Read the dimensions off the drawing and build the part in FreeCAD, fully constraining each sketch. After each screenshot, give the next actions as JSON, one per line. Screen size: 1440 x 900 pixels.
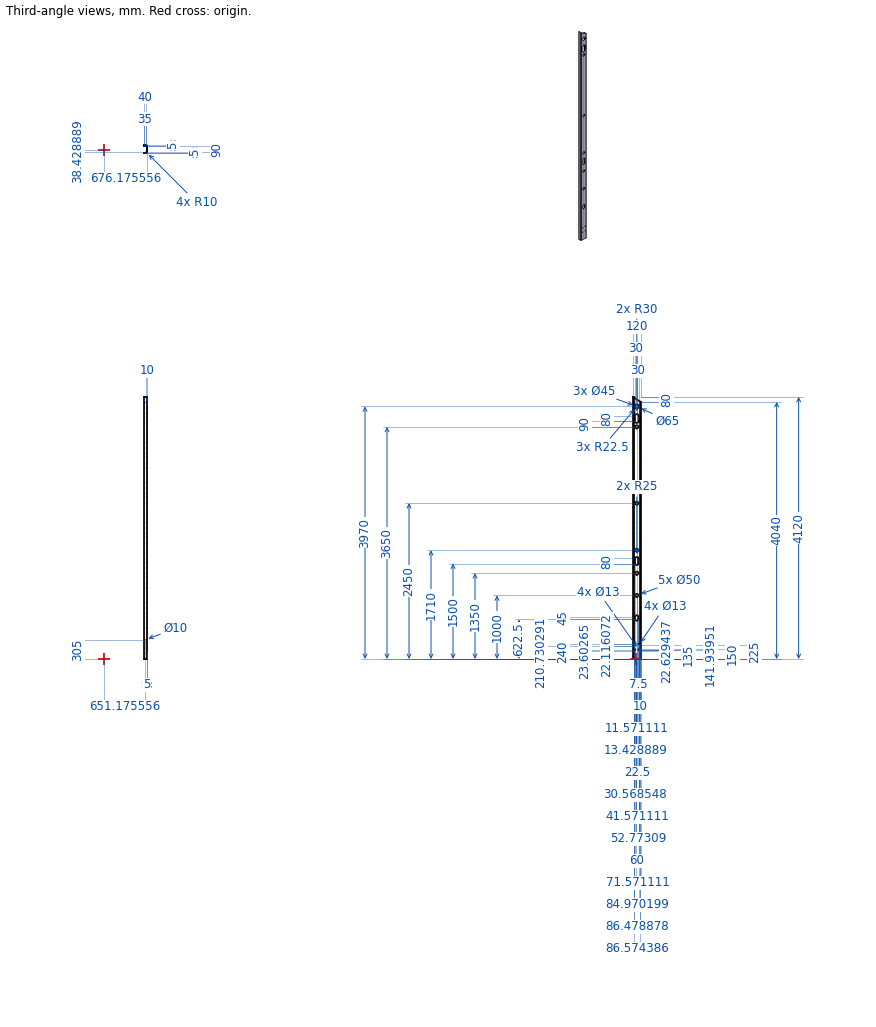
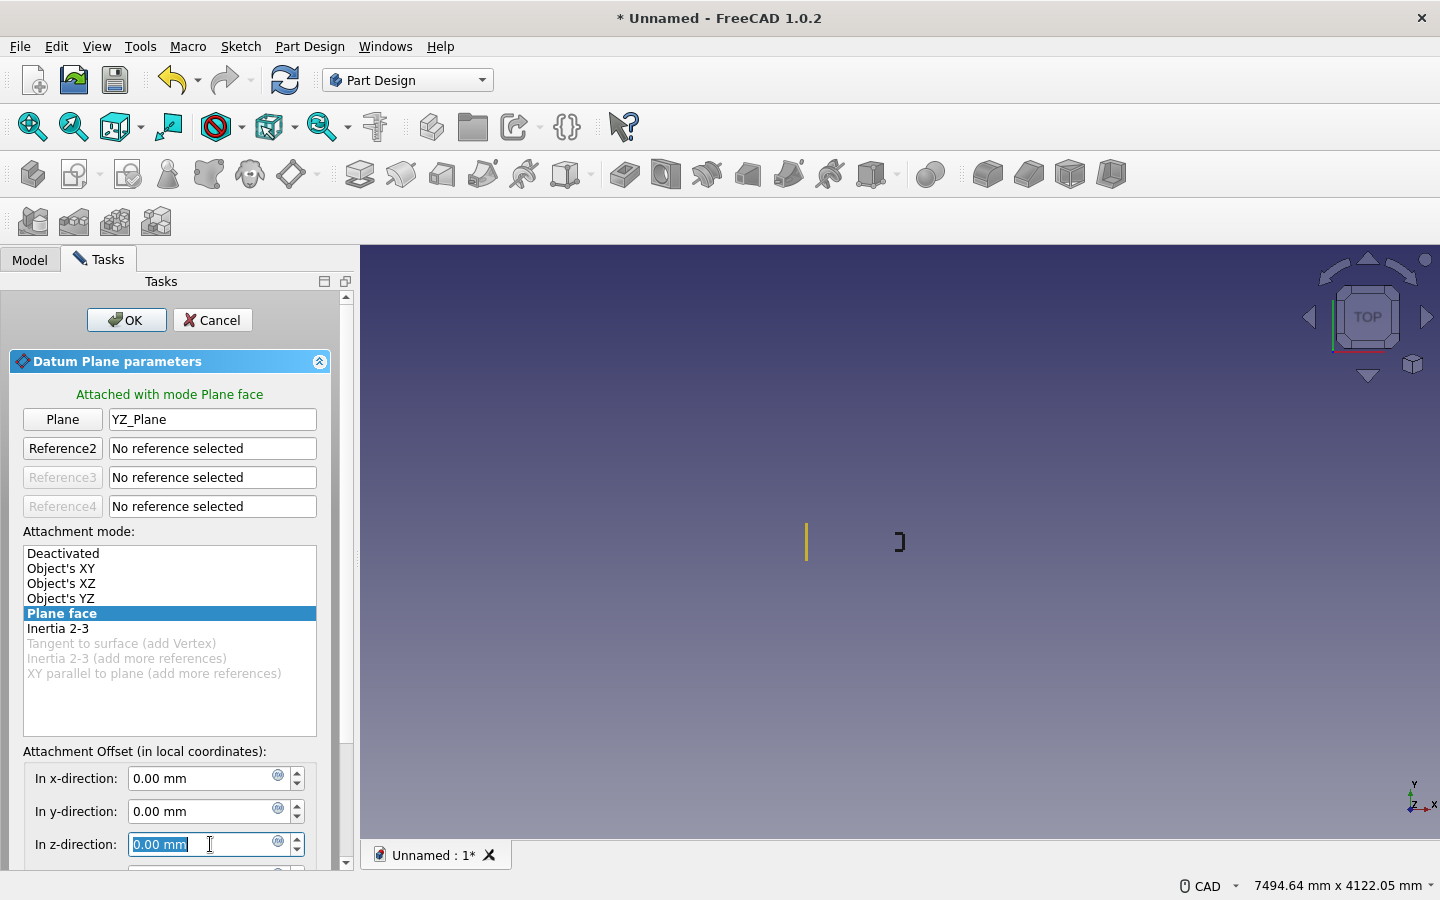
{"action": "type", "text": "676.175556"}
{"action": "key", "text": "Tab"}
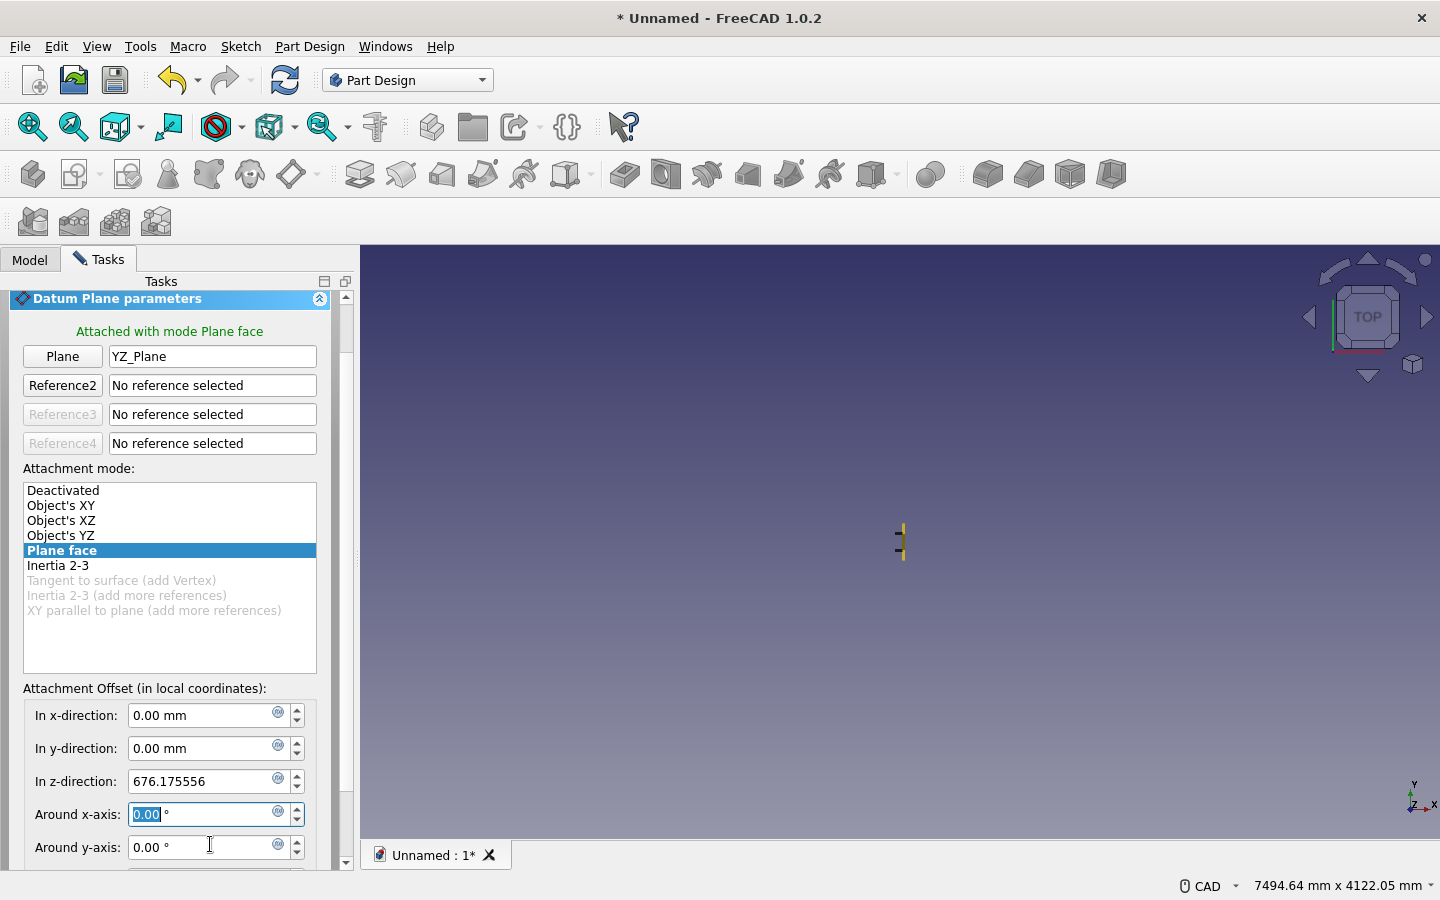
{"action": "scroll", "coordinate": [346, 580], "scroll_direction": "up", "scroll_amount": 2}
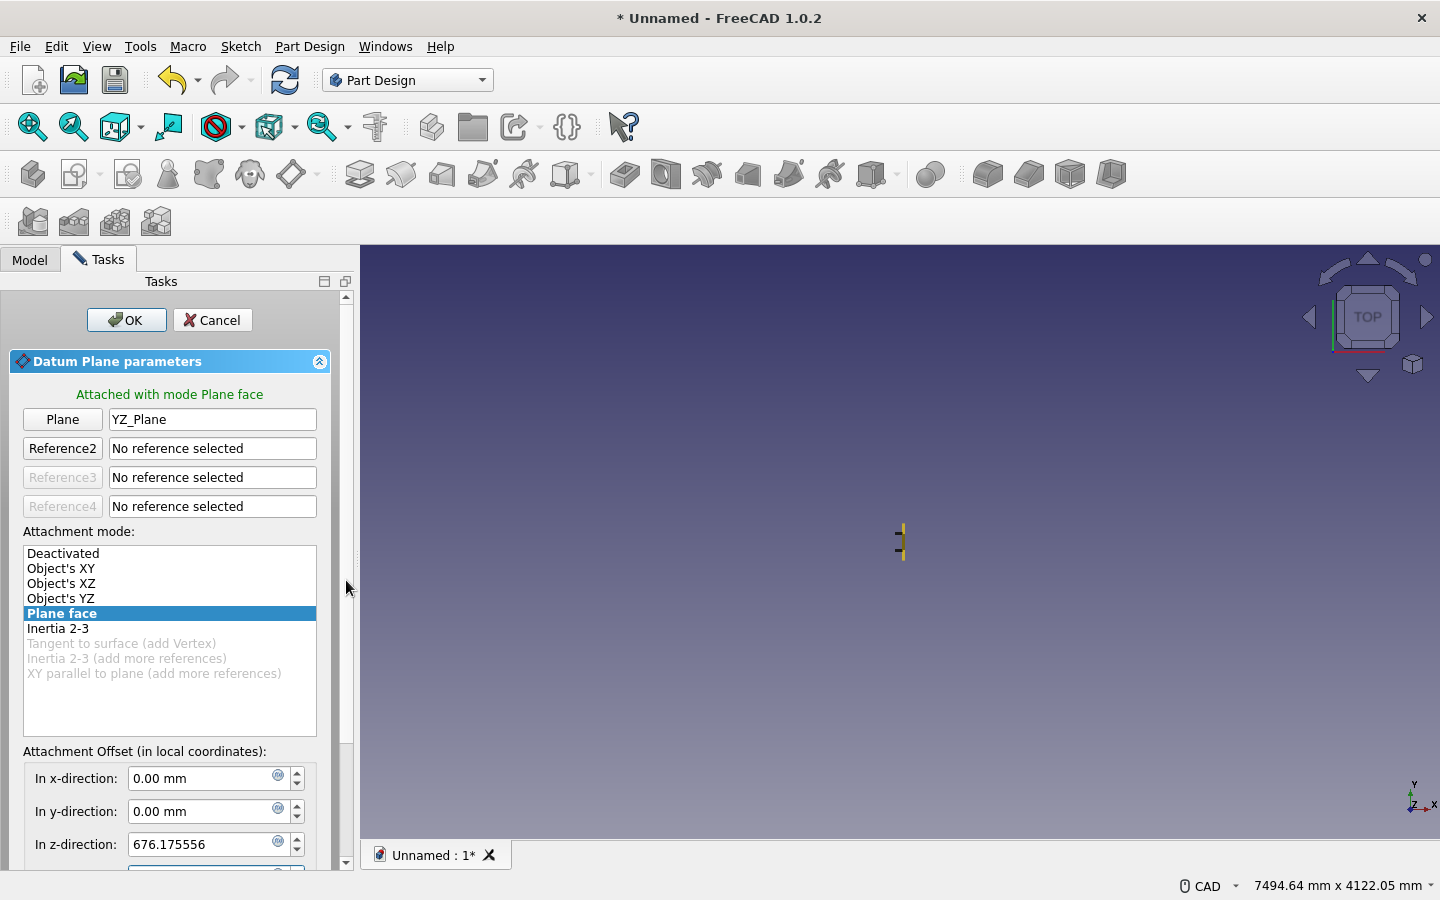
{"action": "left_click", "coordinate": [127, 320]}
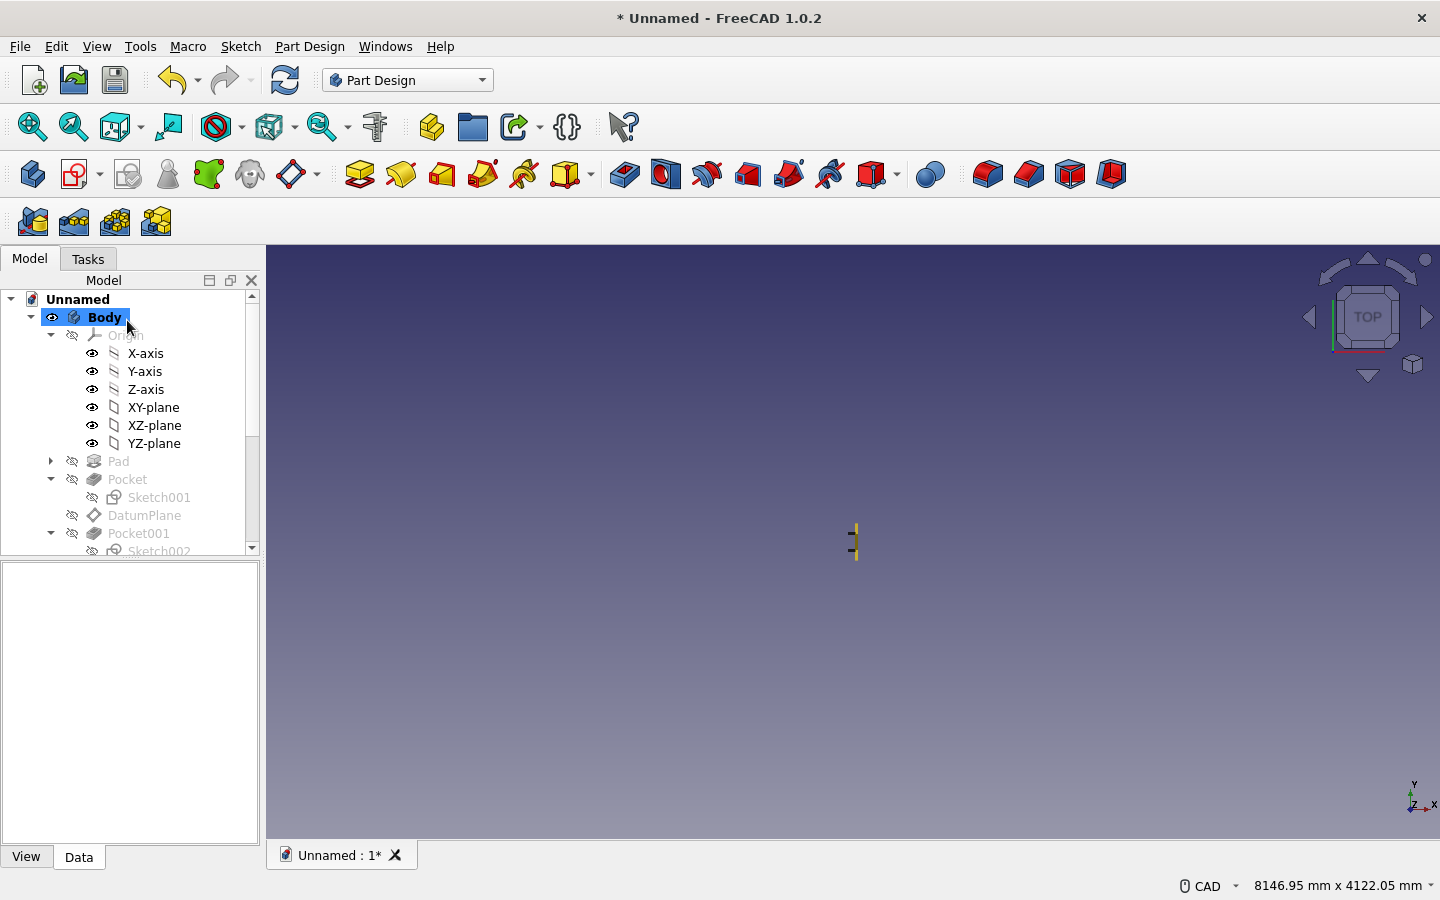
{"action": "scroll", "coordinate": [101, 421], "scroll_direction": "down", "scroll_amount": 3}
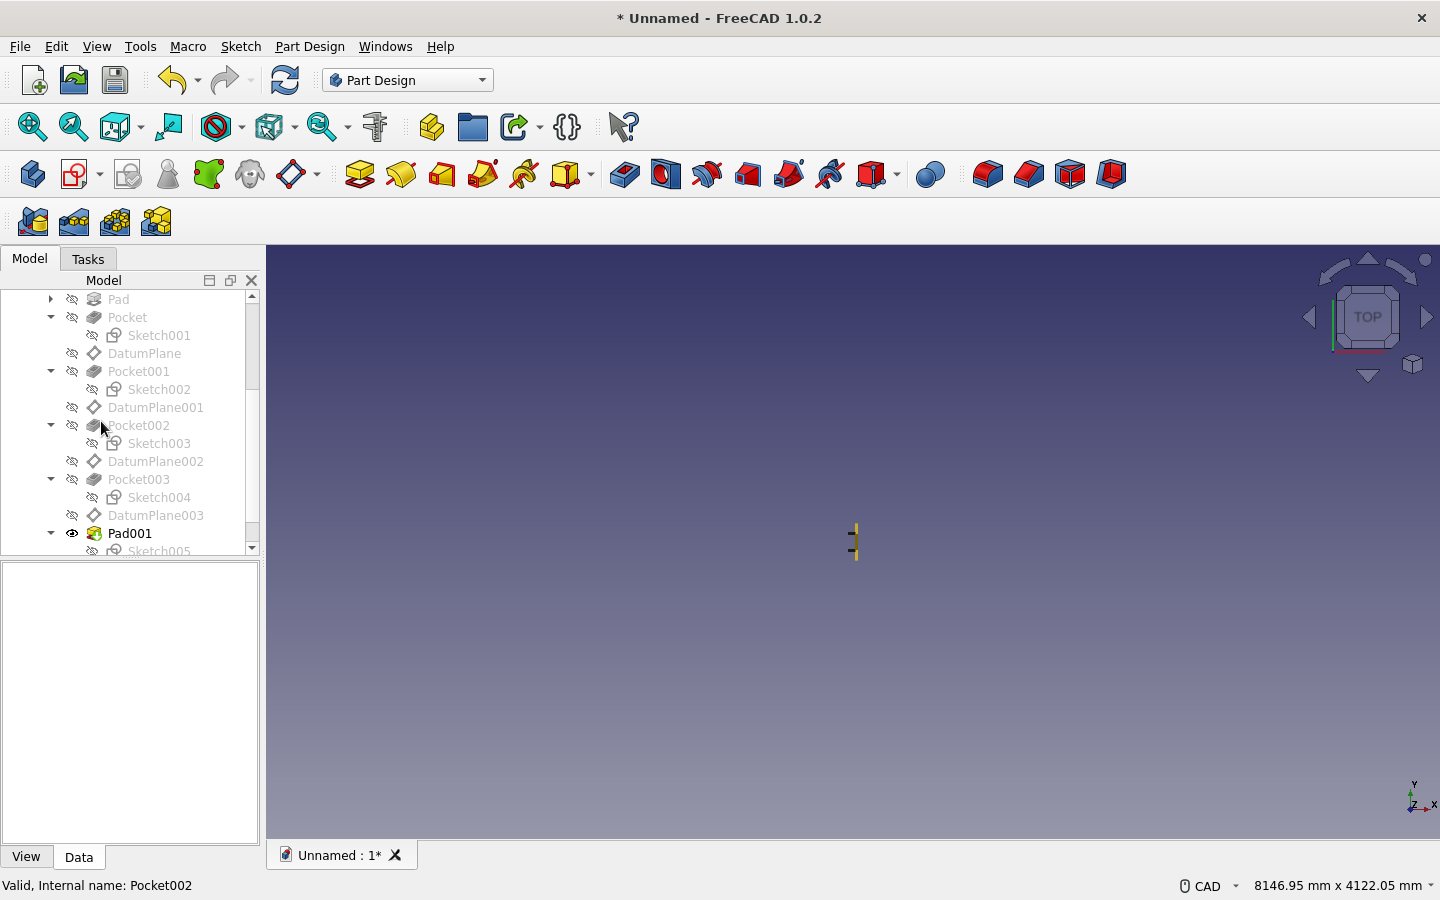
{"action": "scroll", "coordinate": [141, 421], "scroll_direction": "up", "scroll_amount": 15}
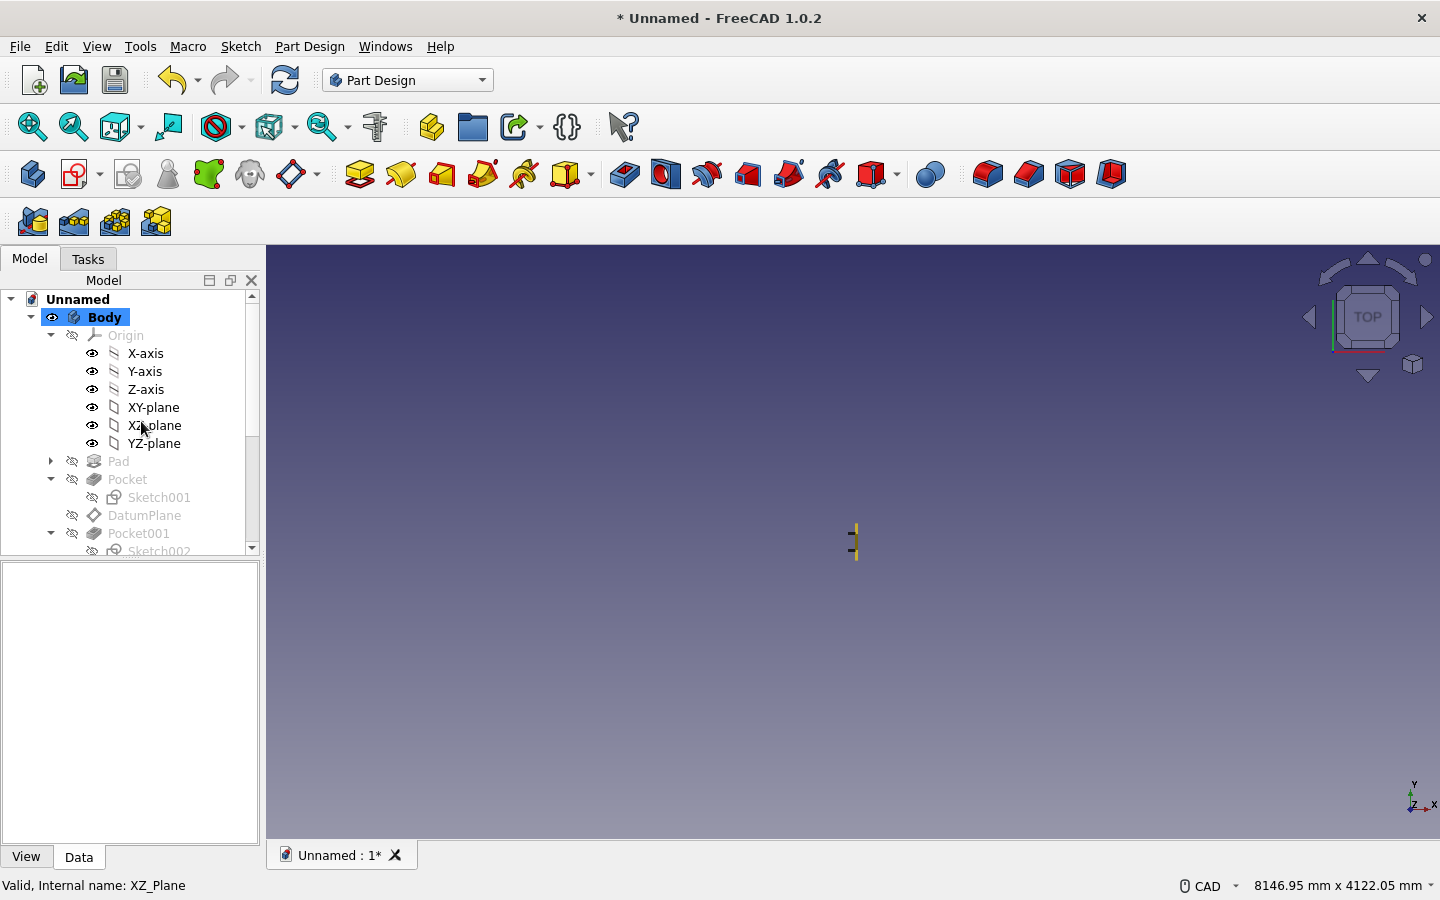
{"action": "scroll", "coordinate": [101, 421], "scroll_direction": "down", "scroll_amount": 6}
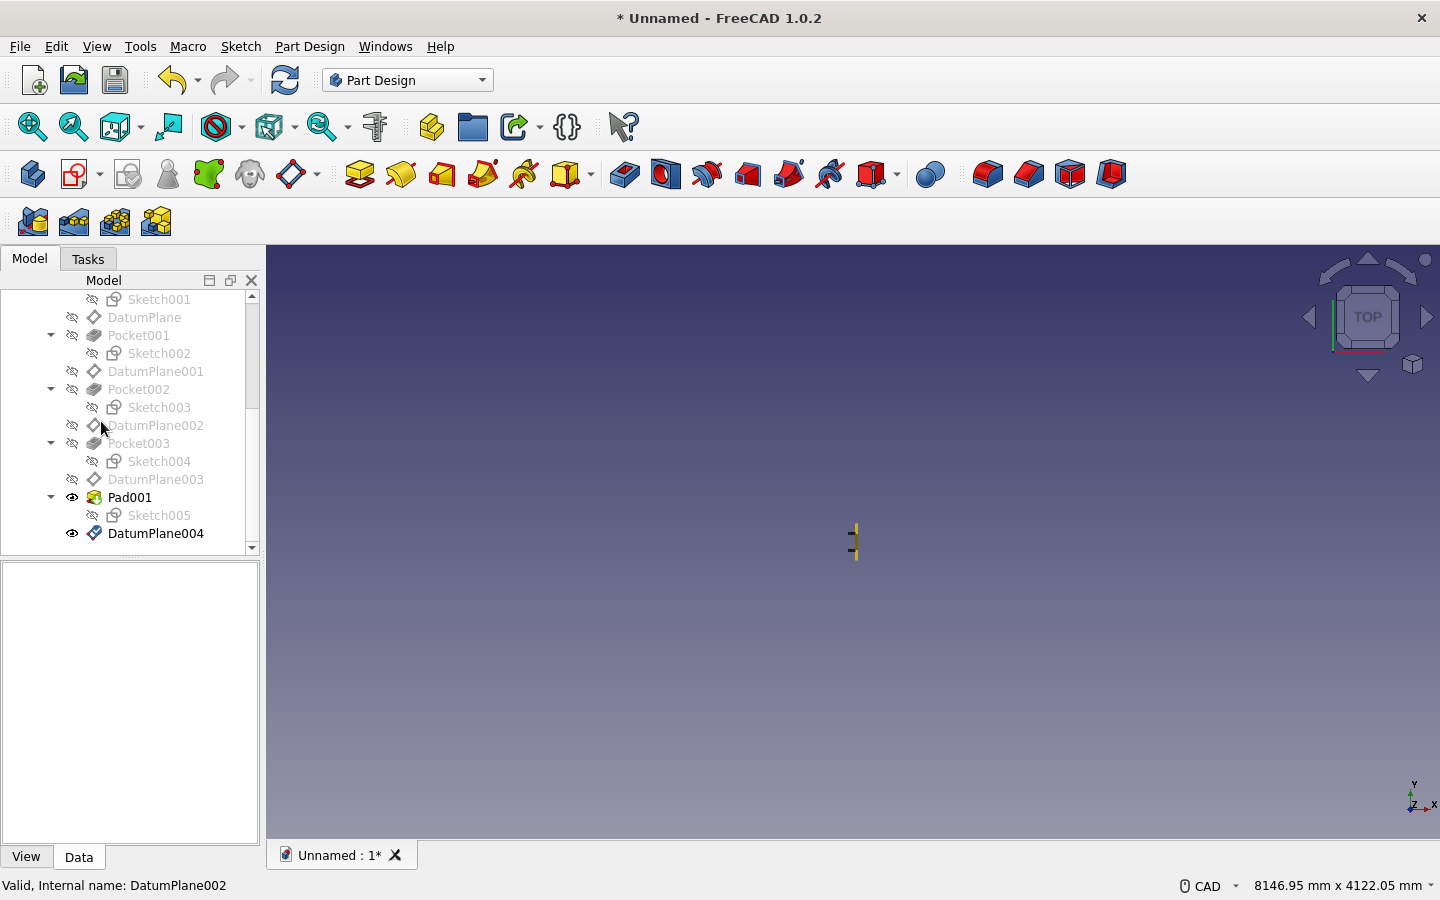
{"action": "left_click", "coordinate": [117, 533]}